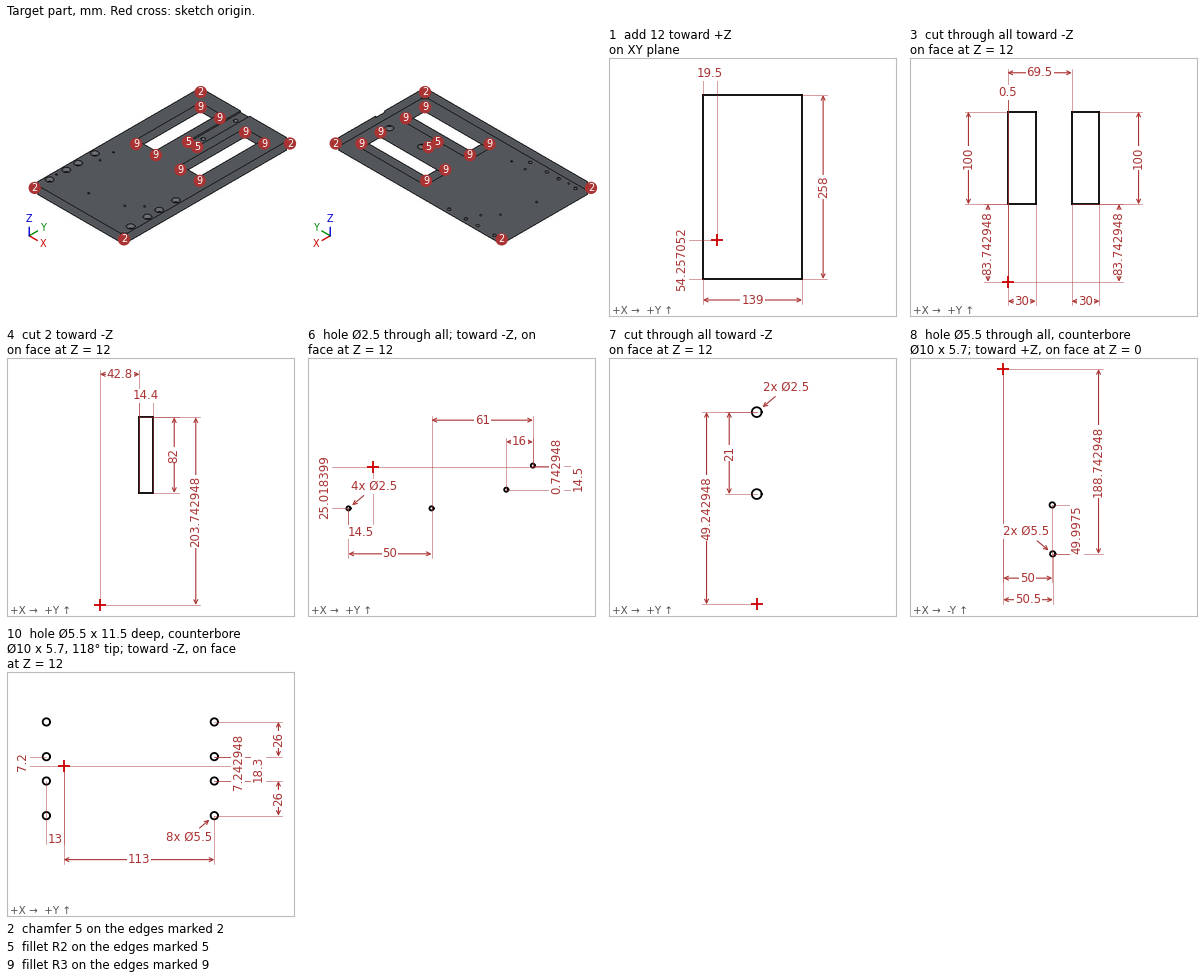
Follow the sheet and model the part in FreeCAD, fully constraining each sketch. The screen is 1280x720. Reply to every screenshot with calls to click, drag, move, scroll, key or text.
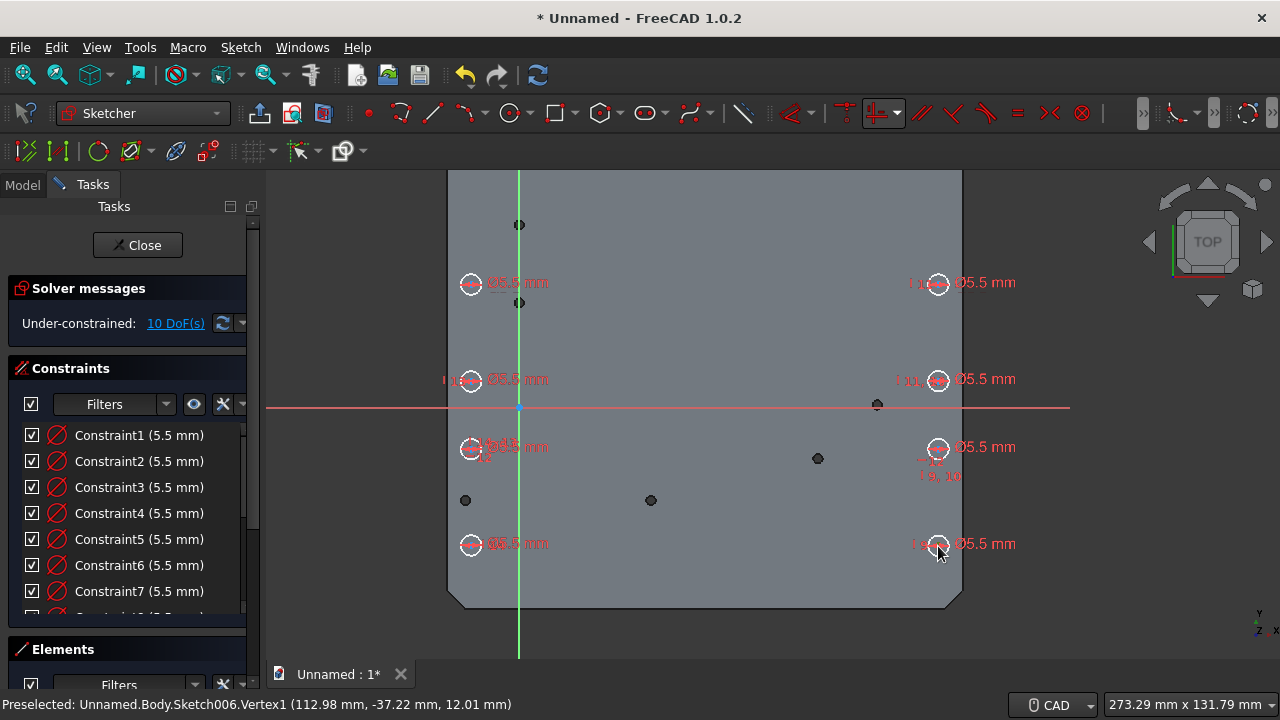
click(471, 545)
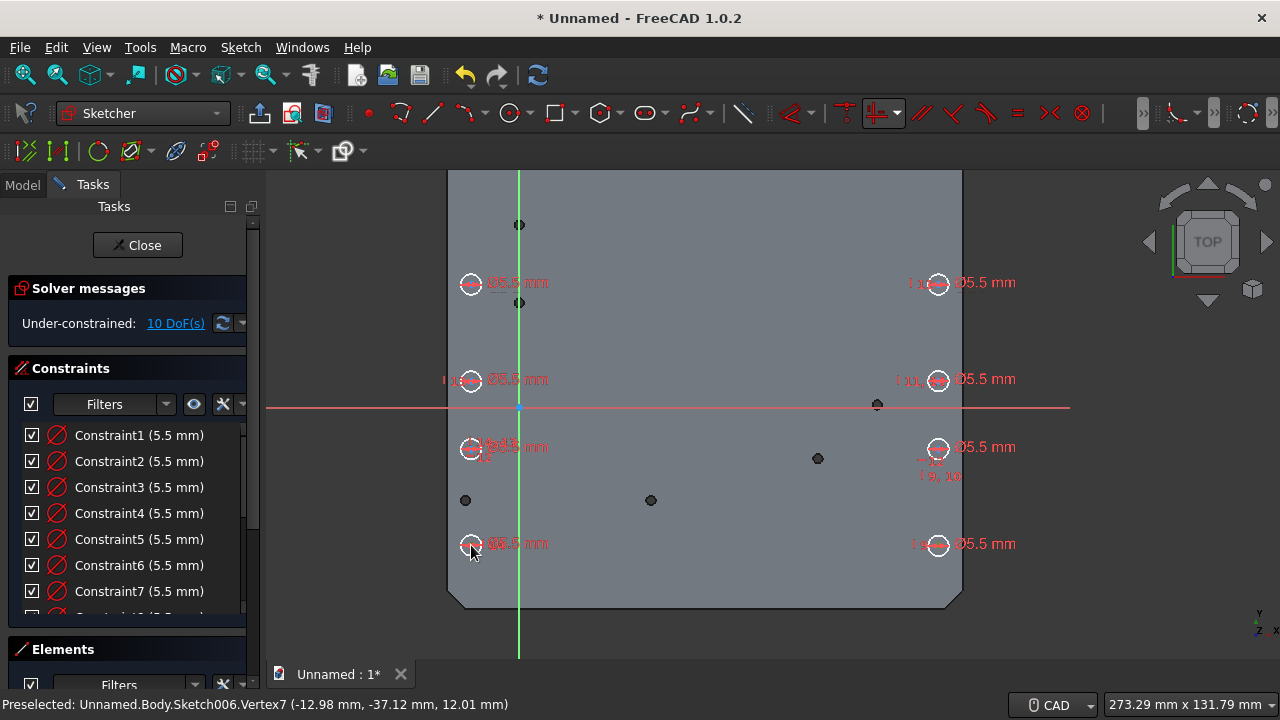
key(h)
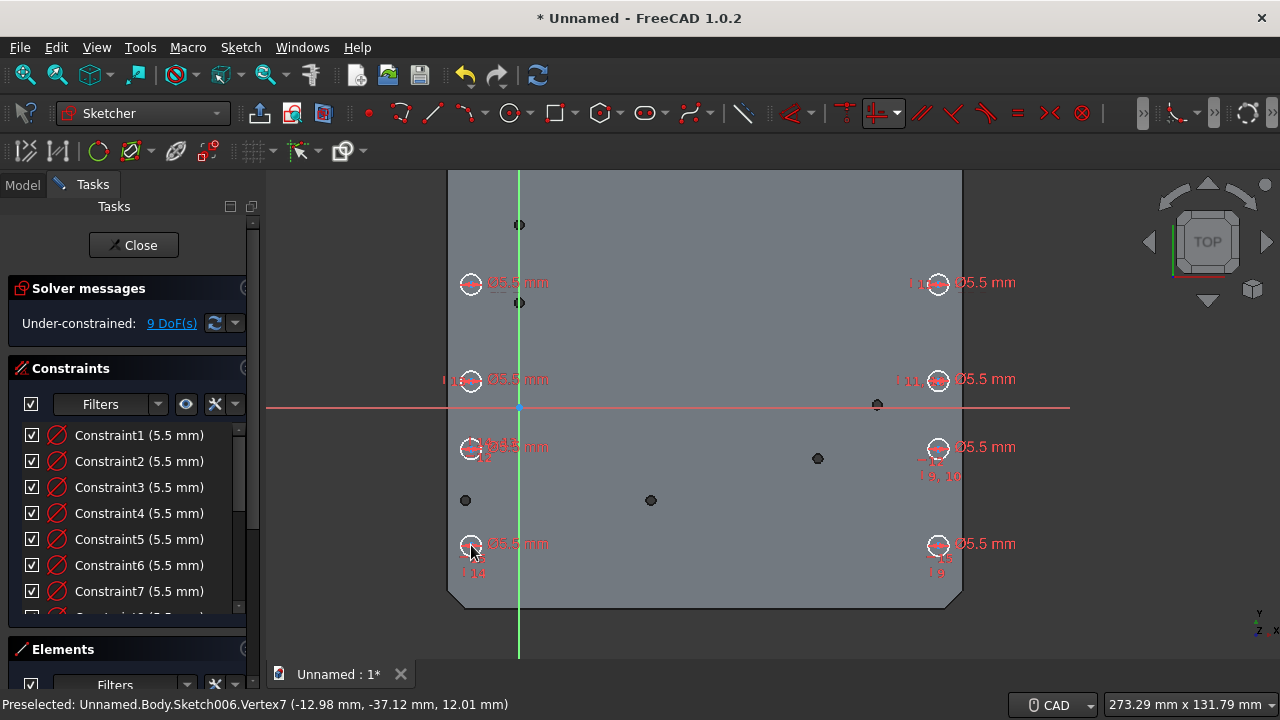
click(471, 381)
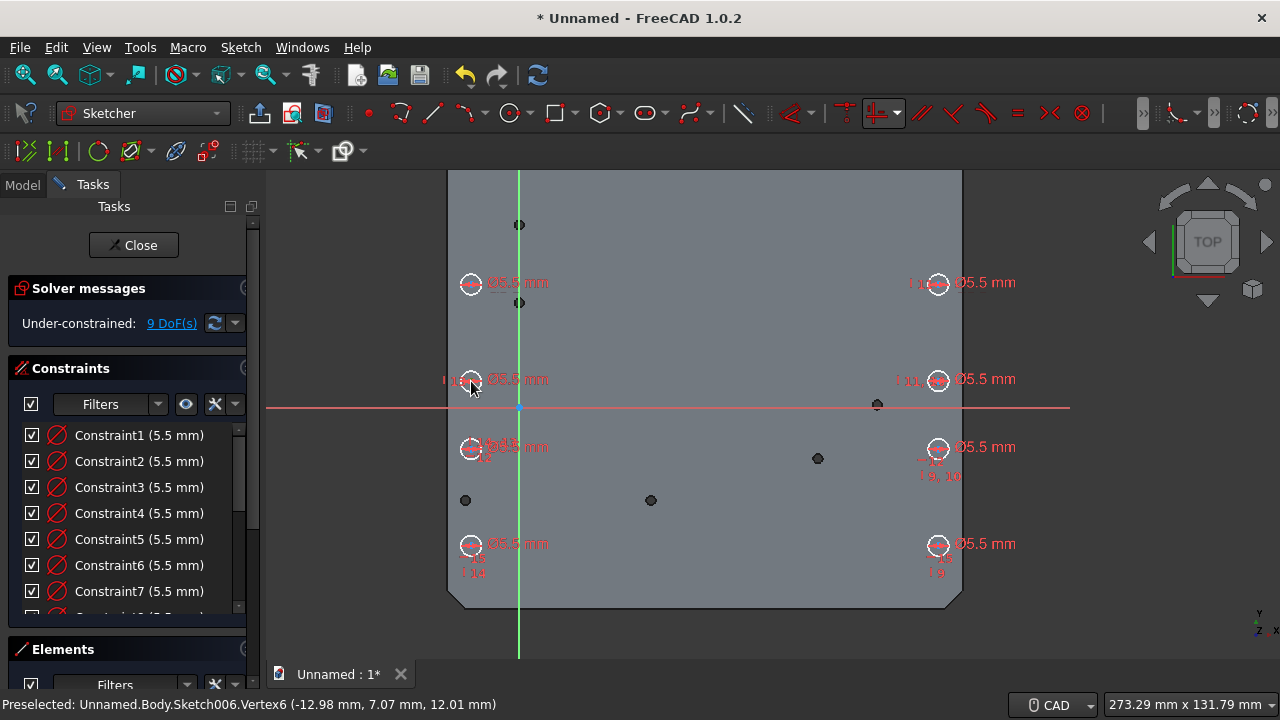
click(471, 285)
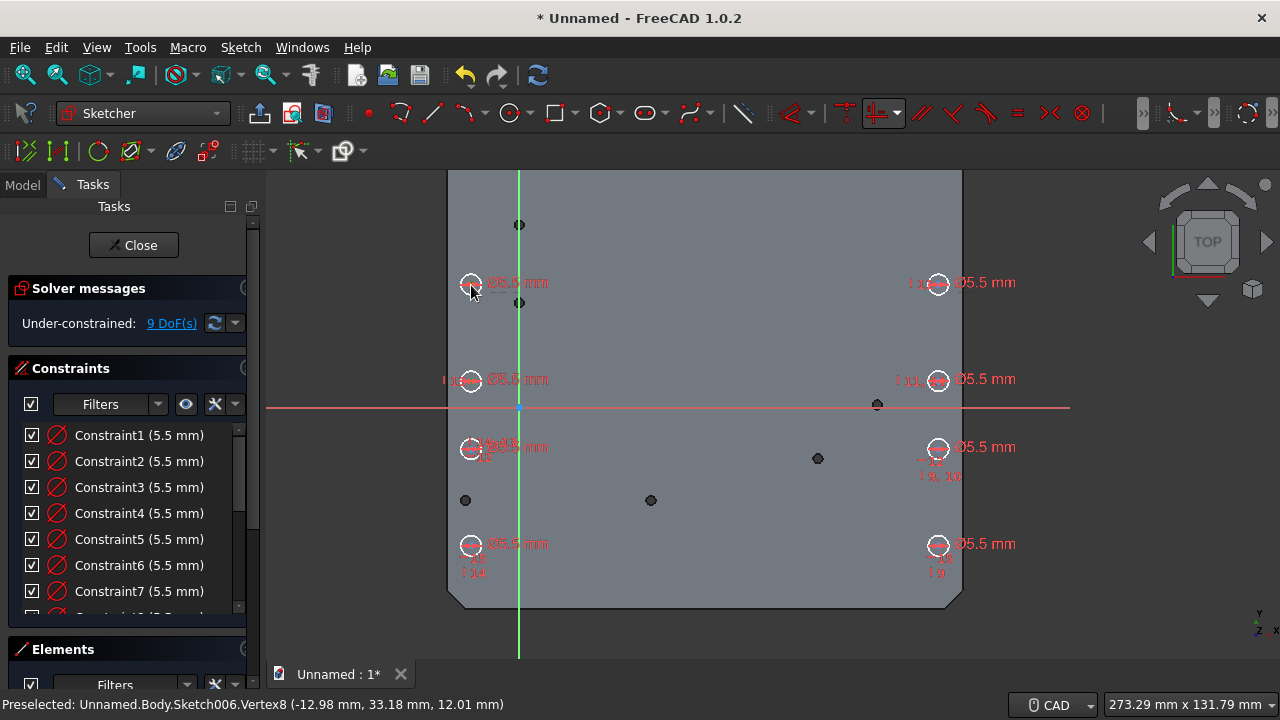
key(v)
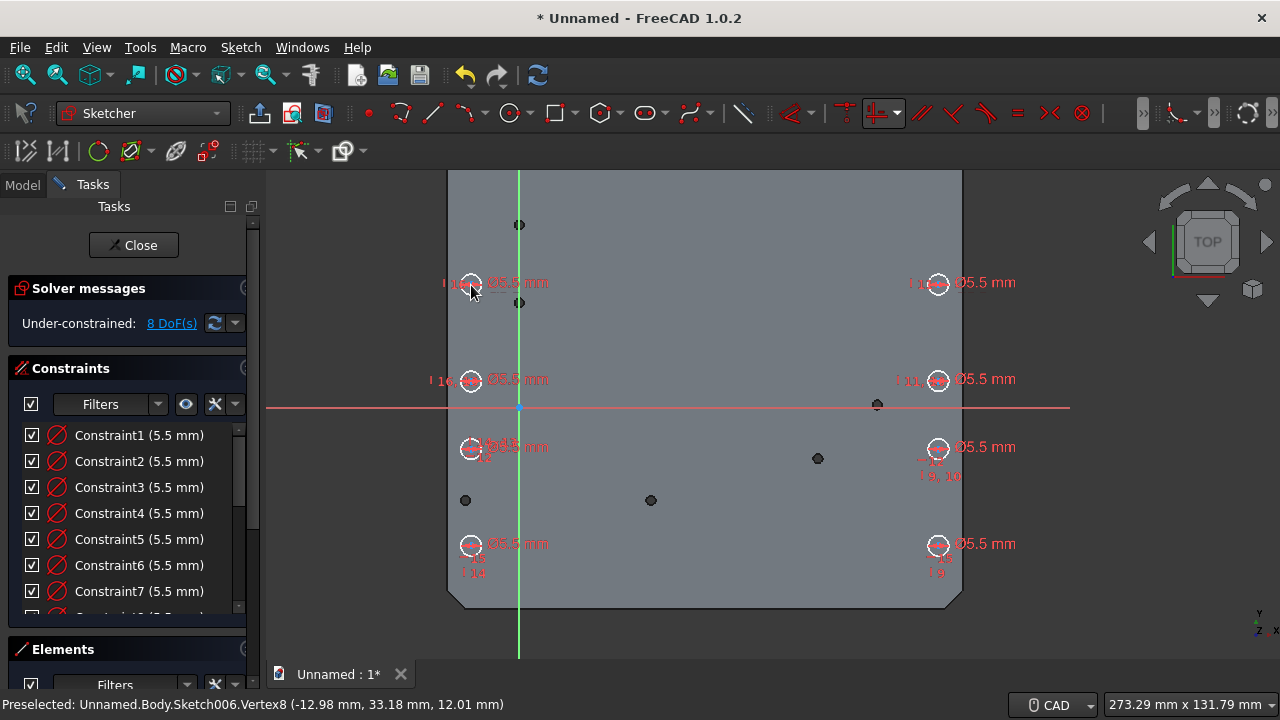
click(938, 285)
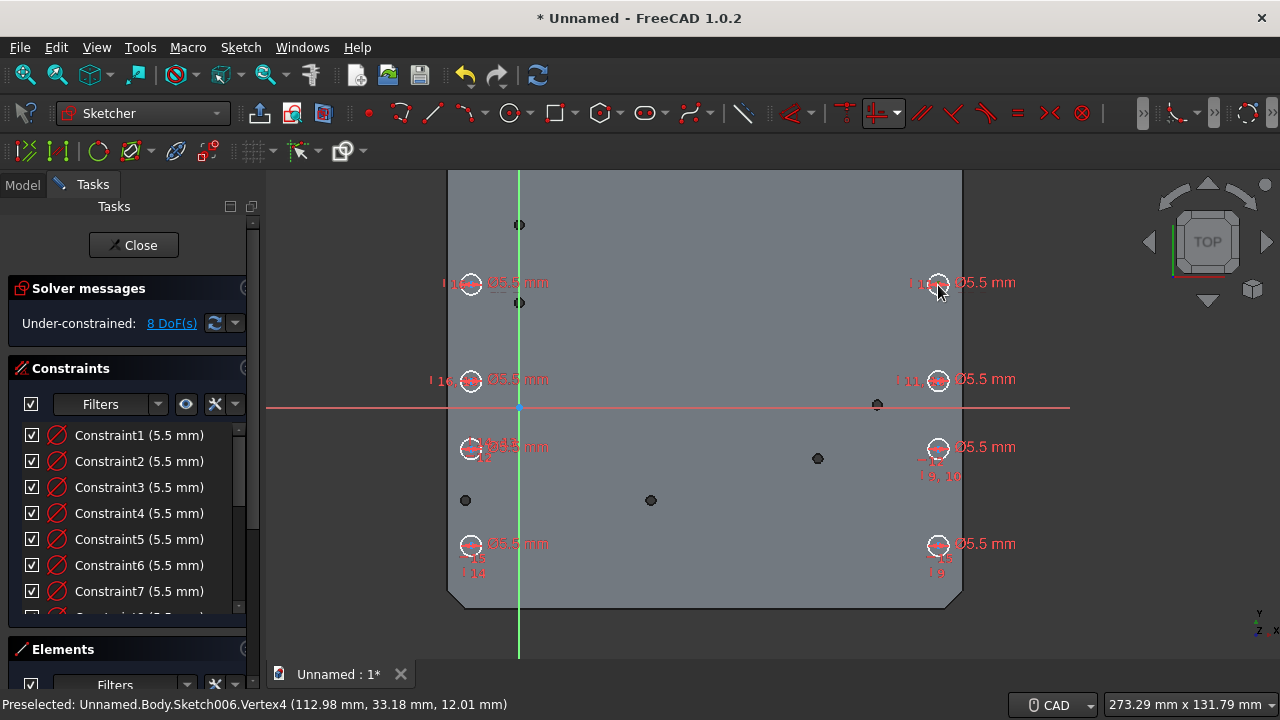
click(471, 285)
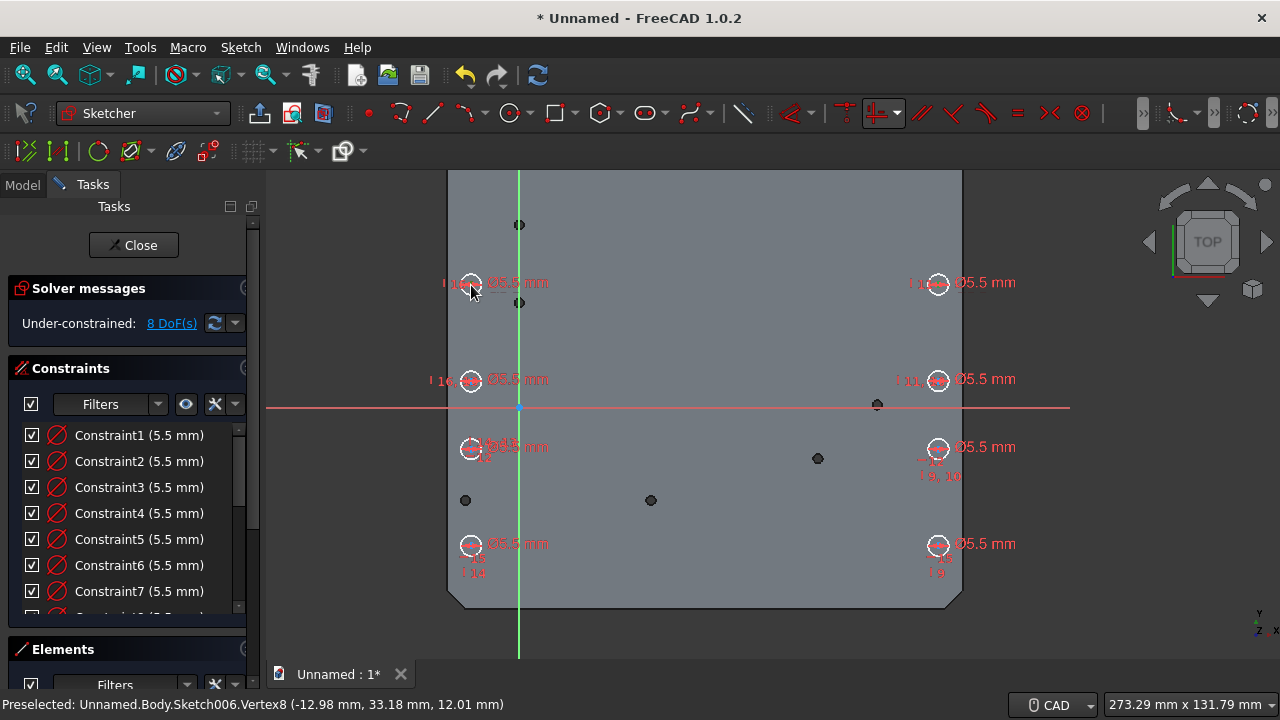
key(h)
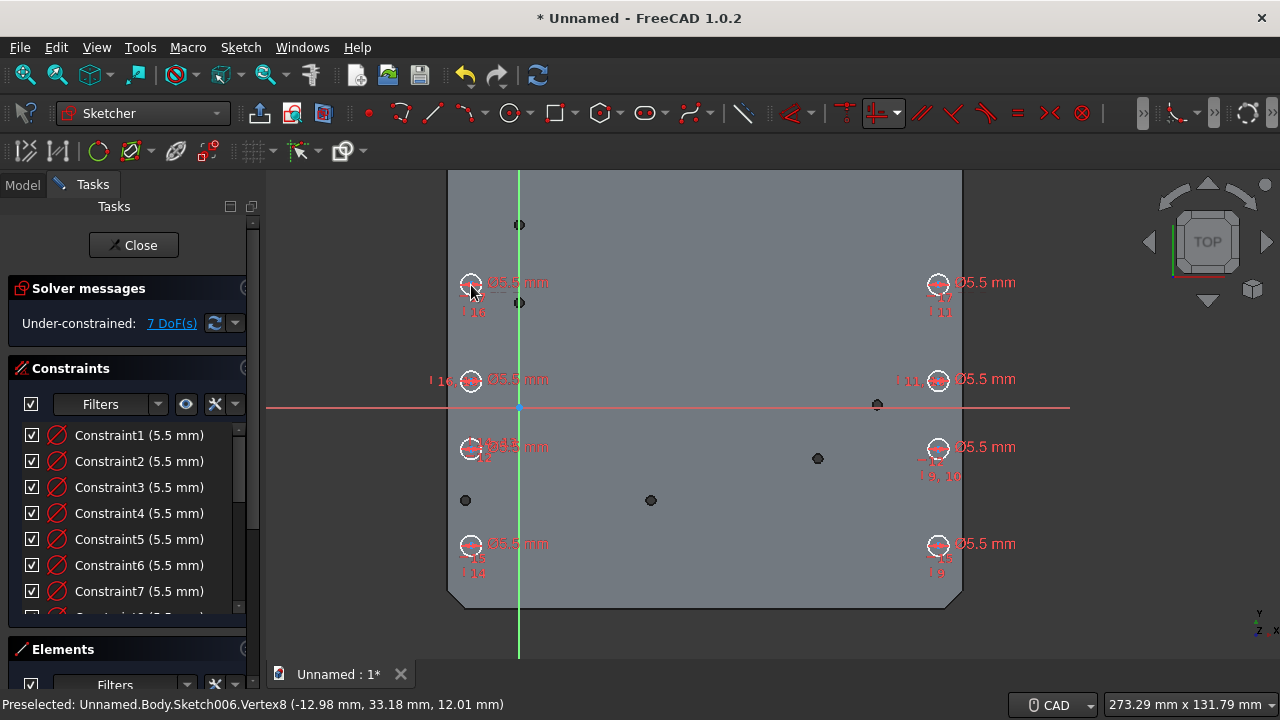
key(d)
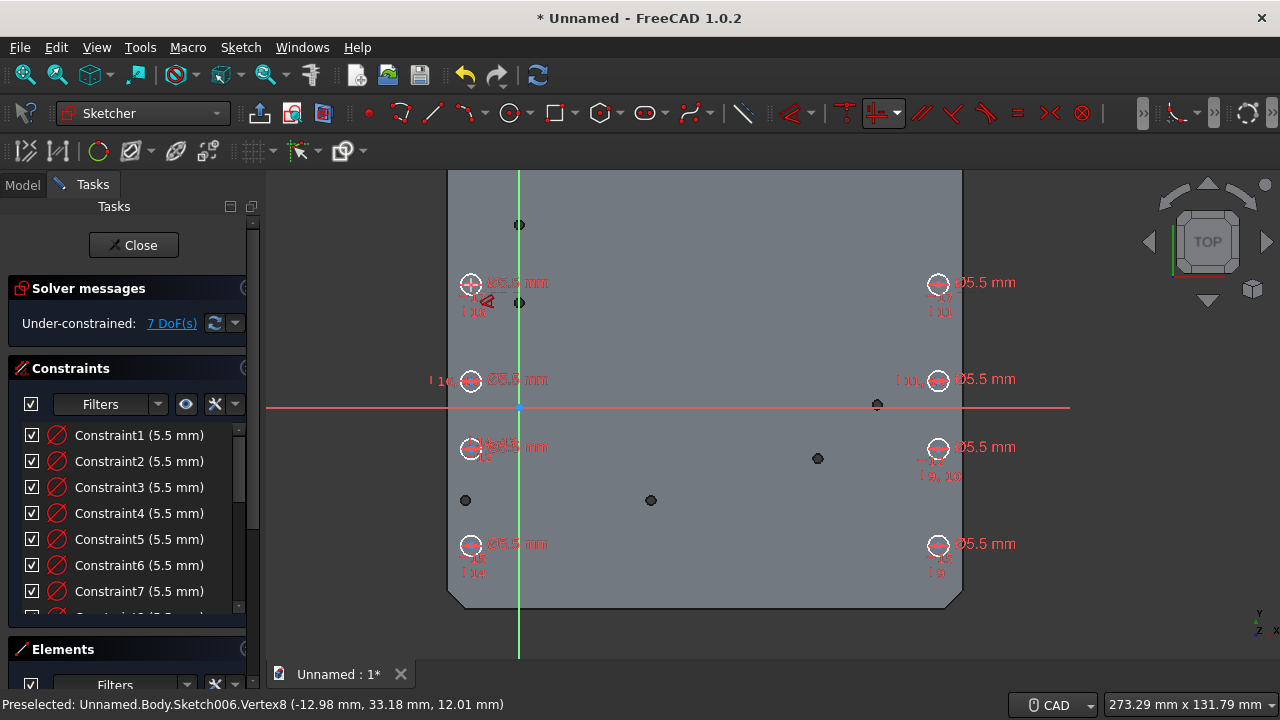
click(471, 449)
click(495, 483)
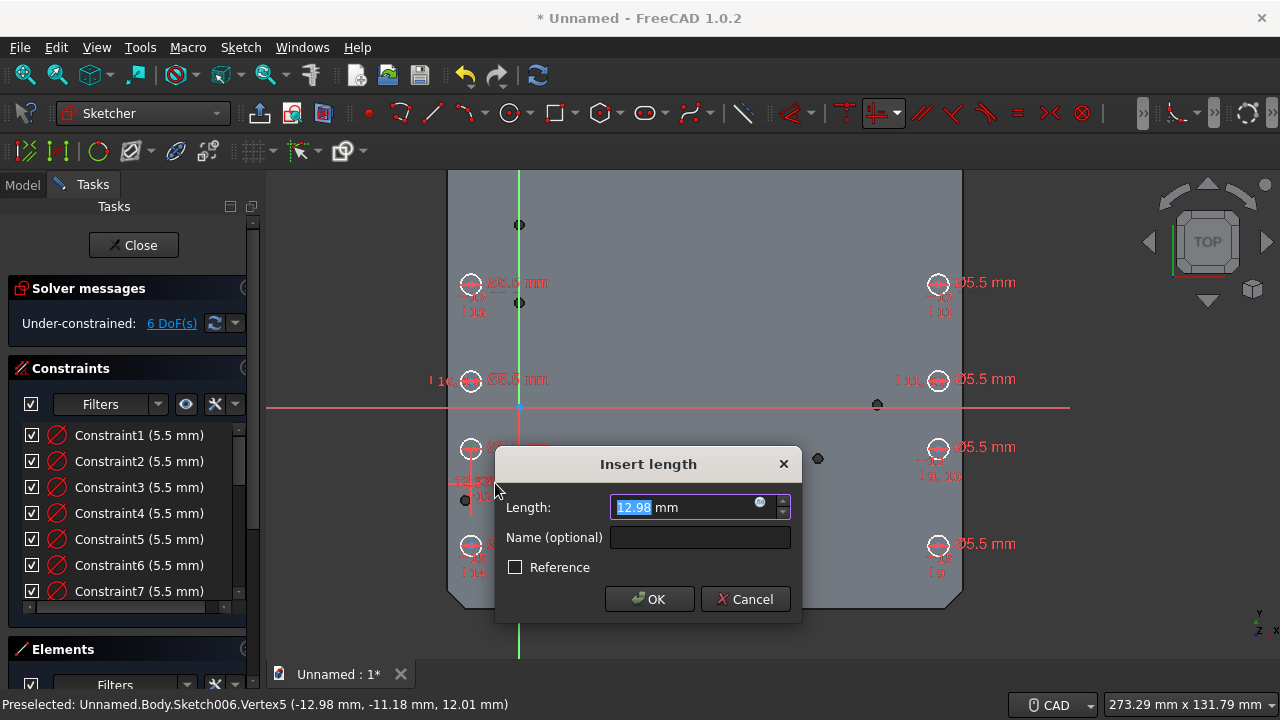
text(13)
key(Return)